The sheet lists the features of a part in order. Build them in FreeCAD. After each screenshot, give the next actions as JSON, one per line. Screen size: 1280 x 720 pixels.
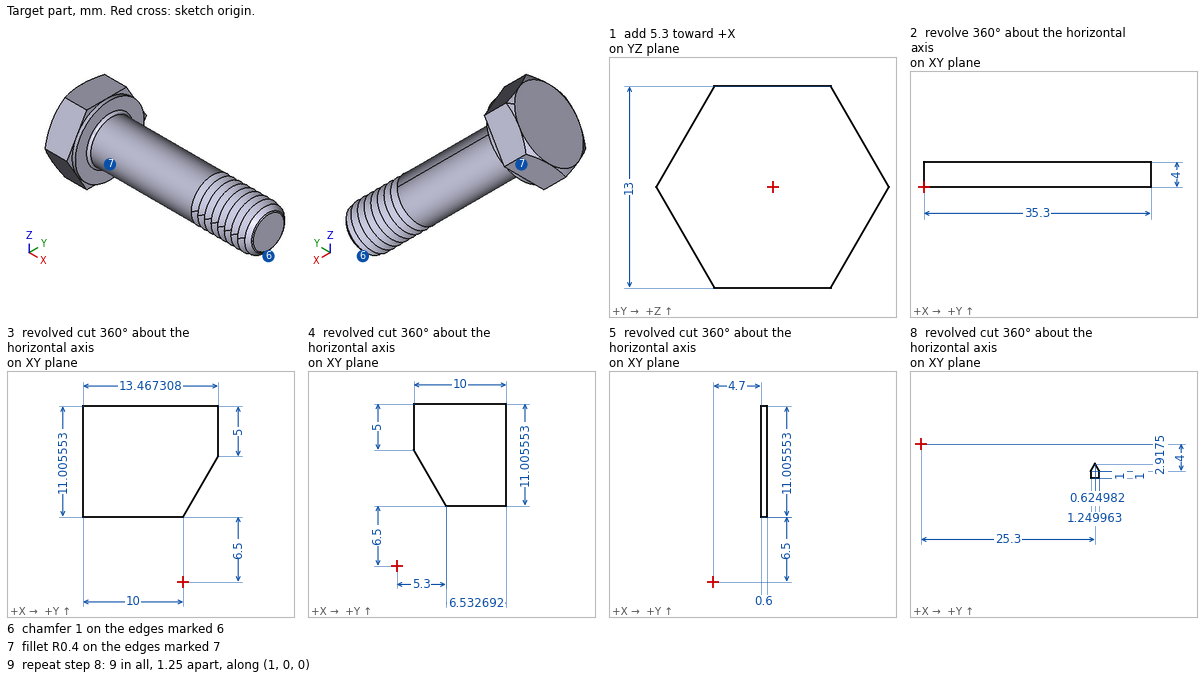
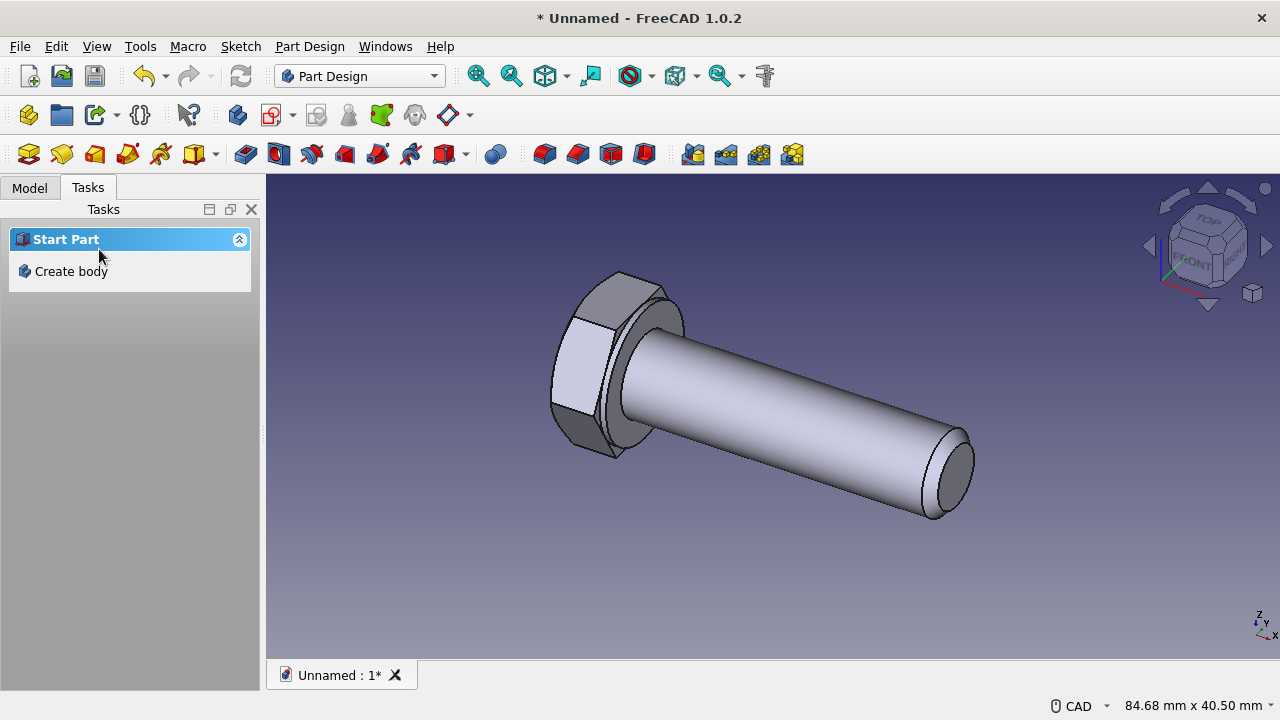
{"action": "key", "text": "0"}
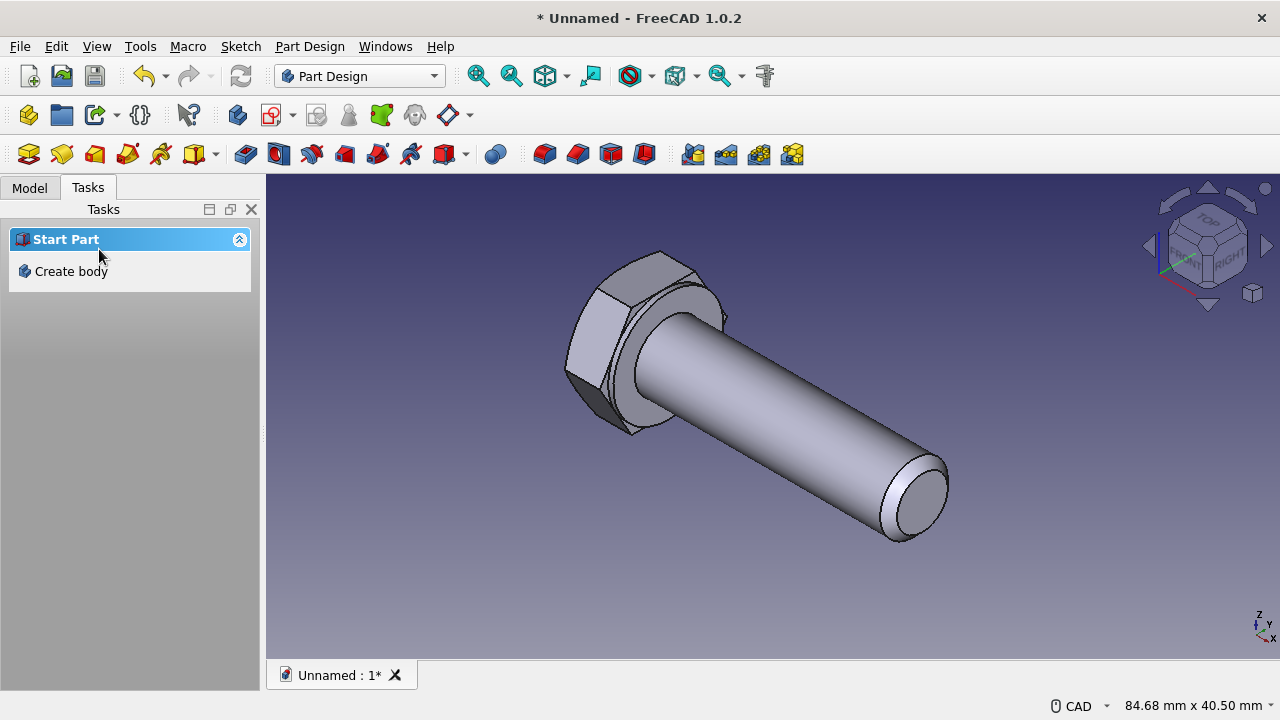
{"action": "key", "text": "2"}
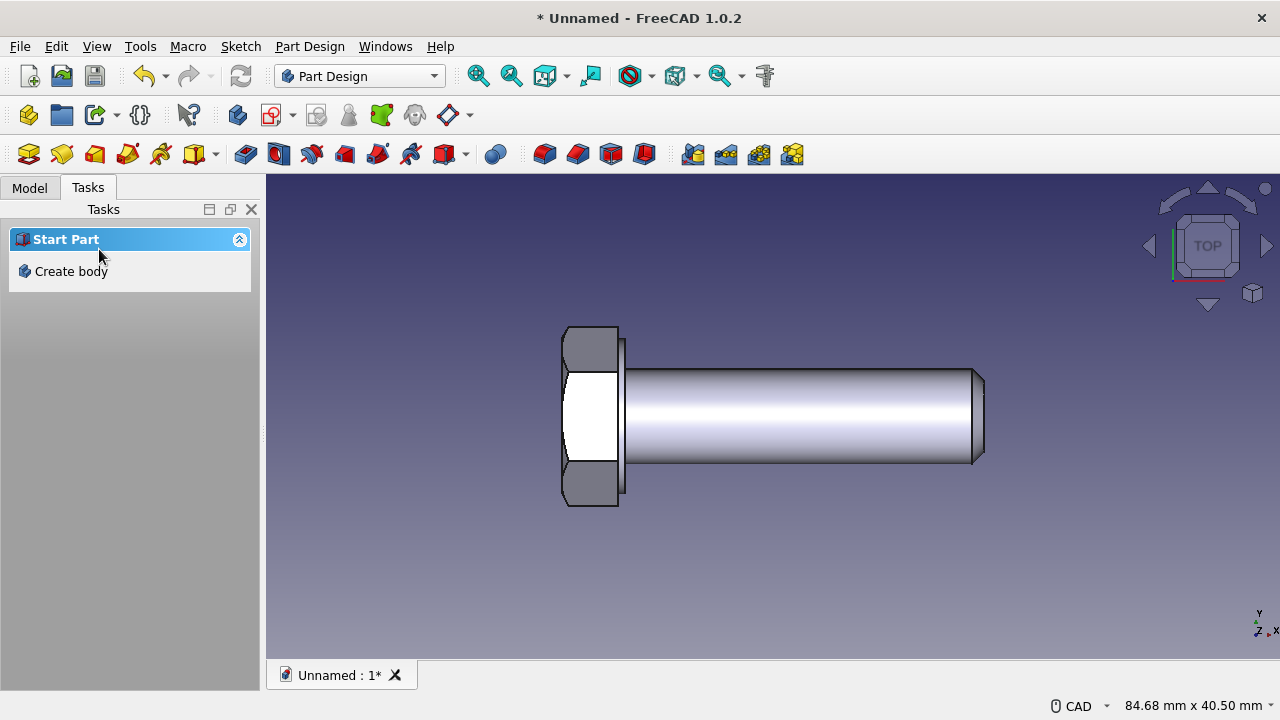
{"action": "left_click", "coordinate": [479, 76]}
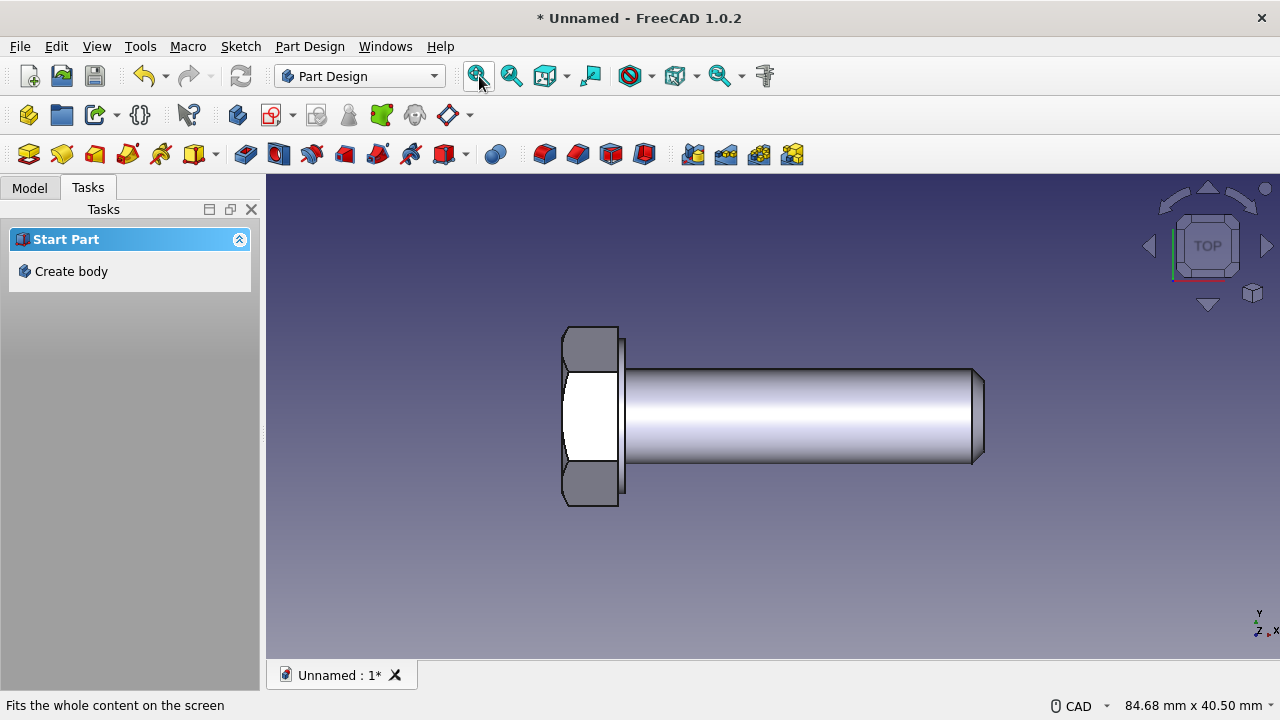
{"action": "key", "text": "1"}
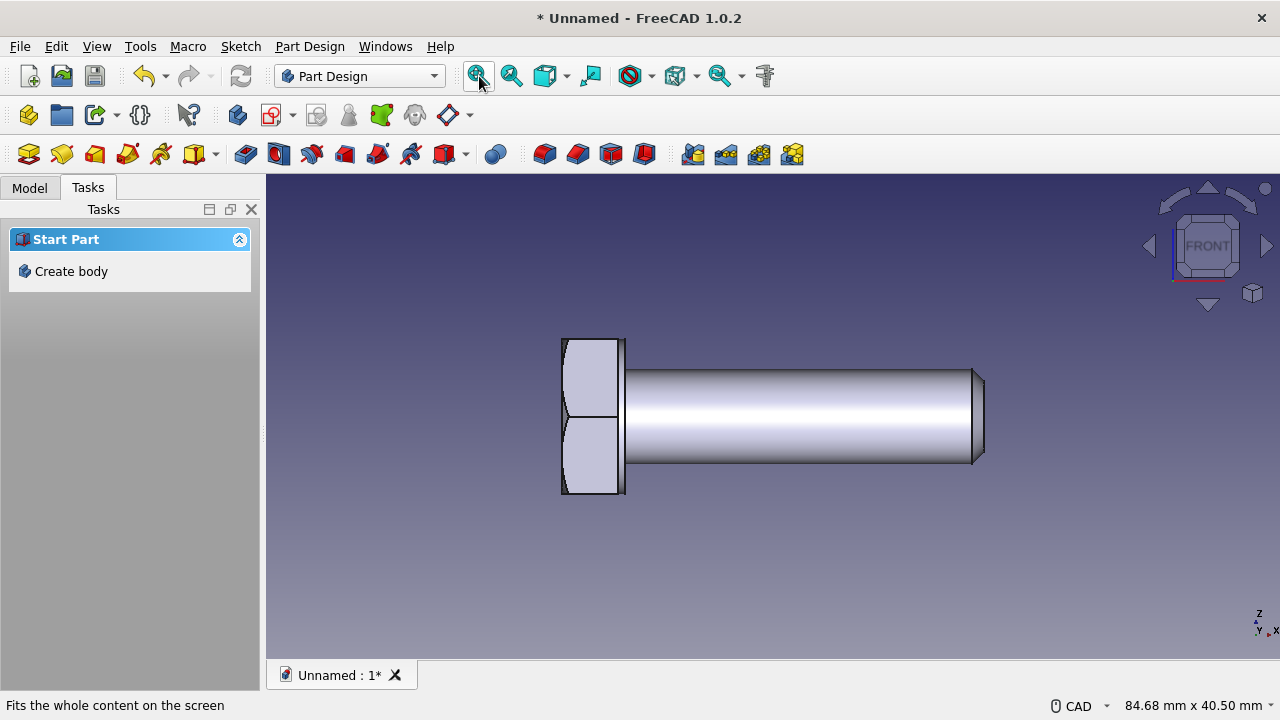
{"action": "left_click", "coordinate": [479, 76]}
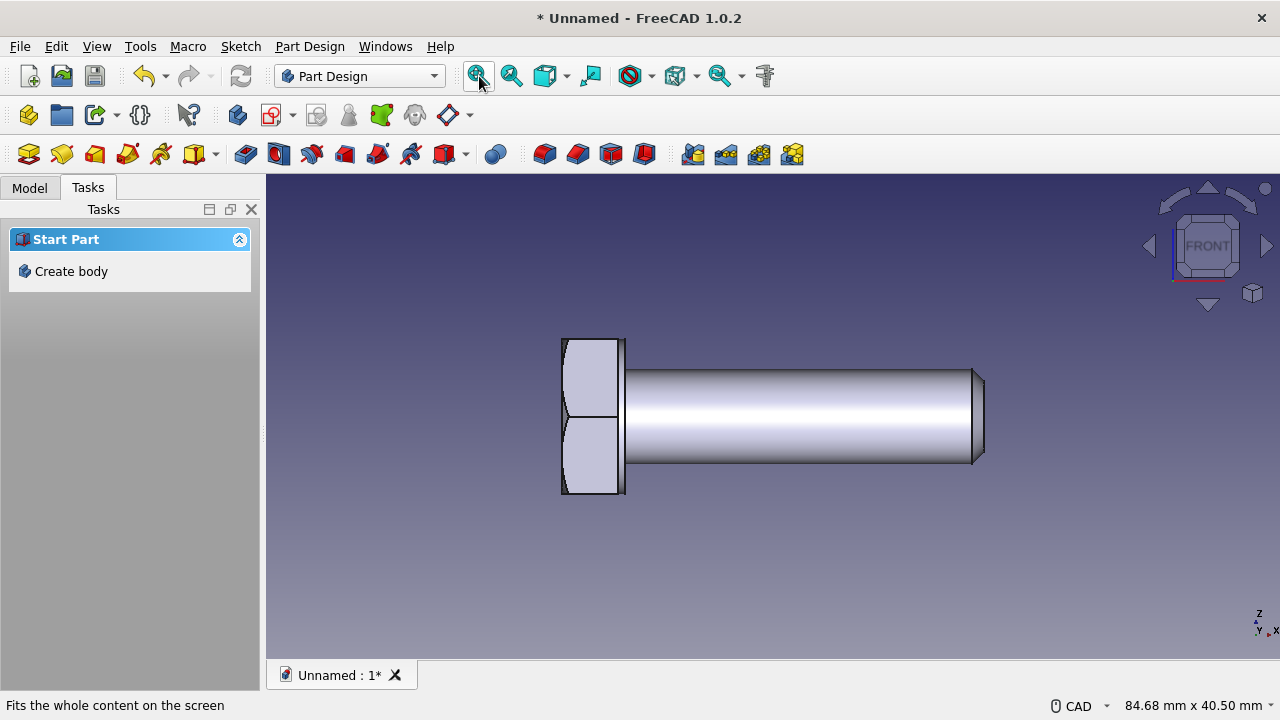
{"action": "key", "text": "3"}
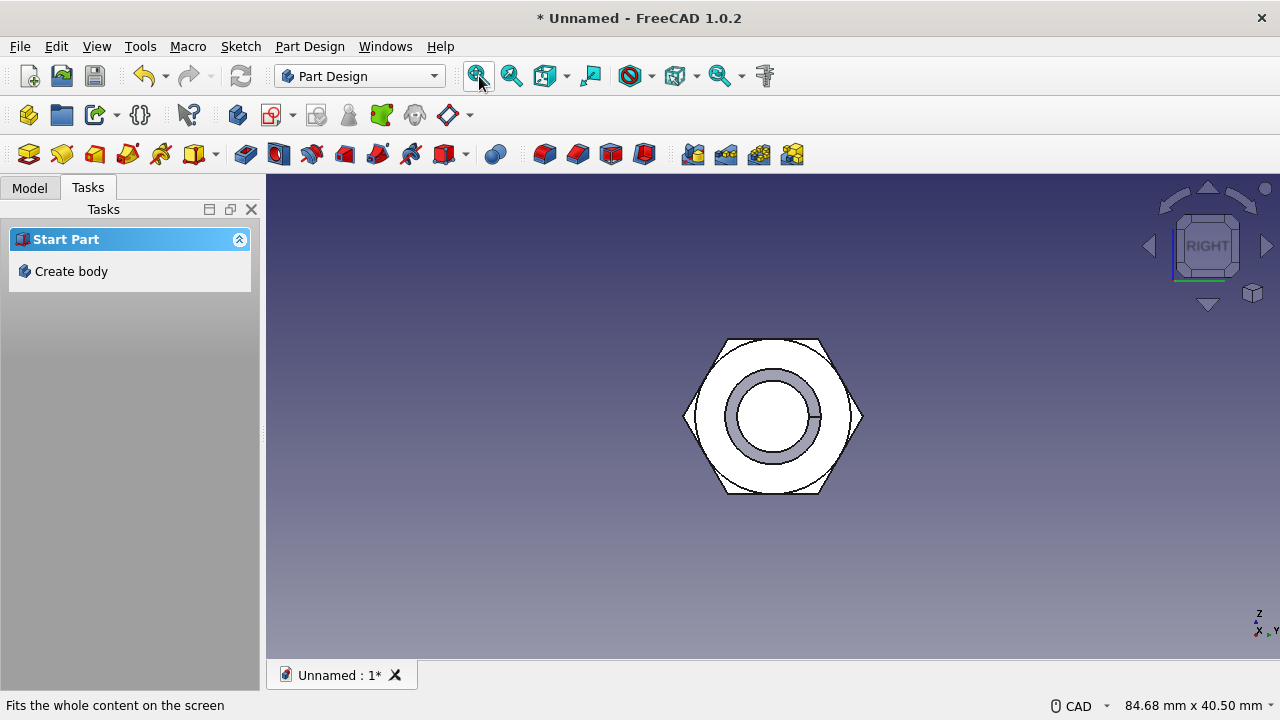
{"action": "left_click", "coordinate": [479, 76]}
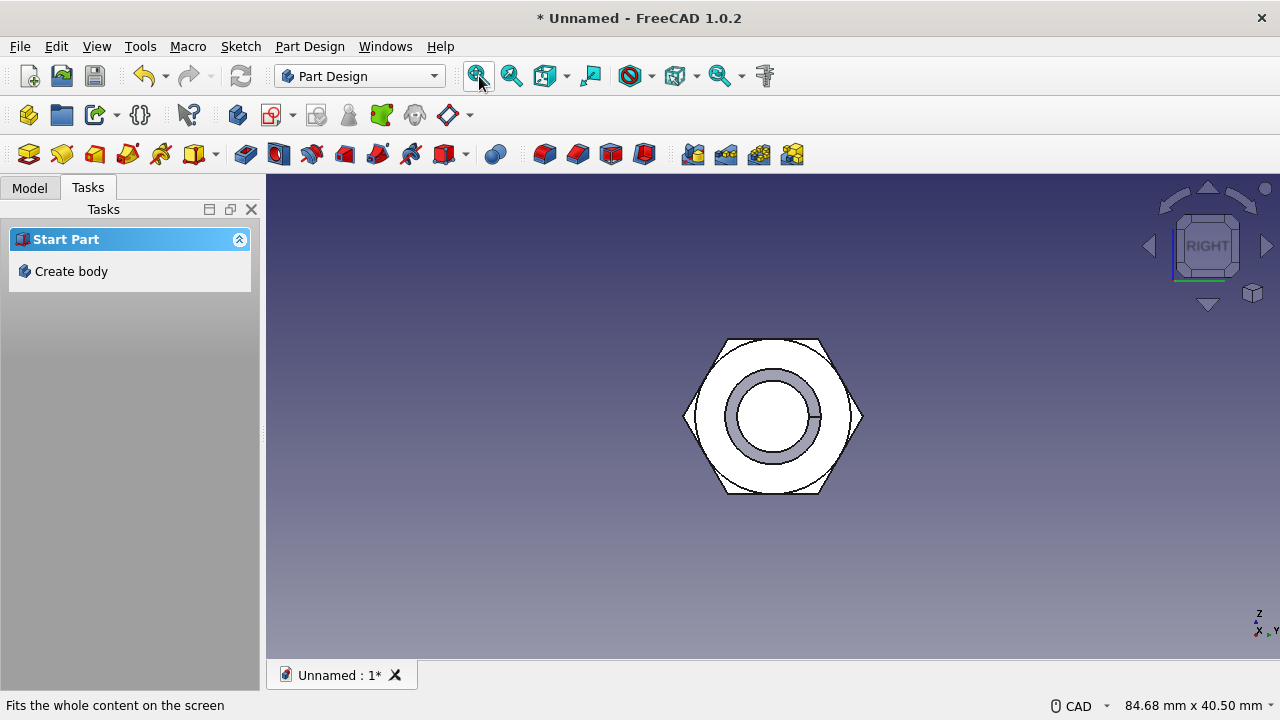
{"action": "key", "text": "5"}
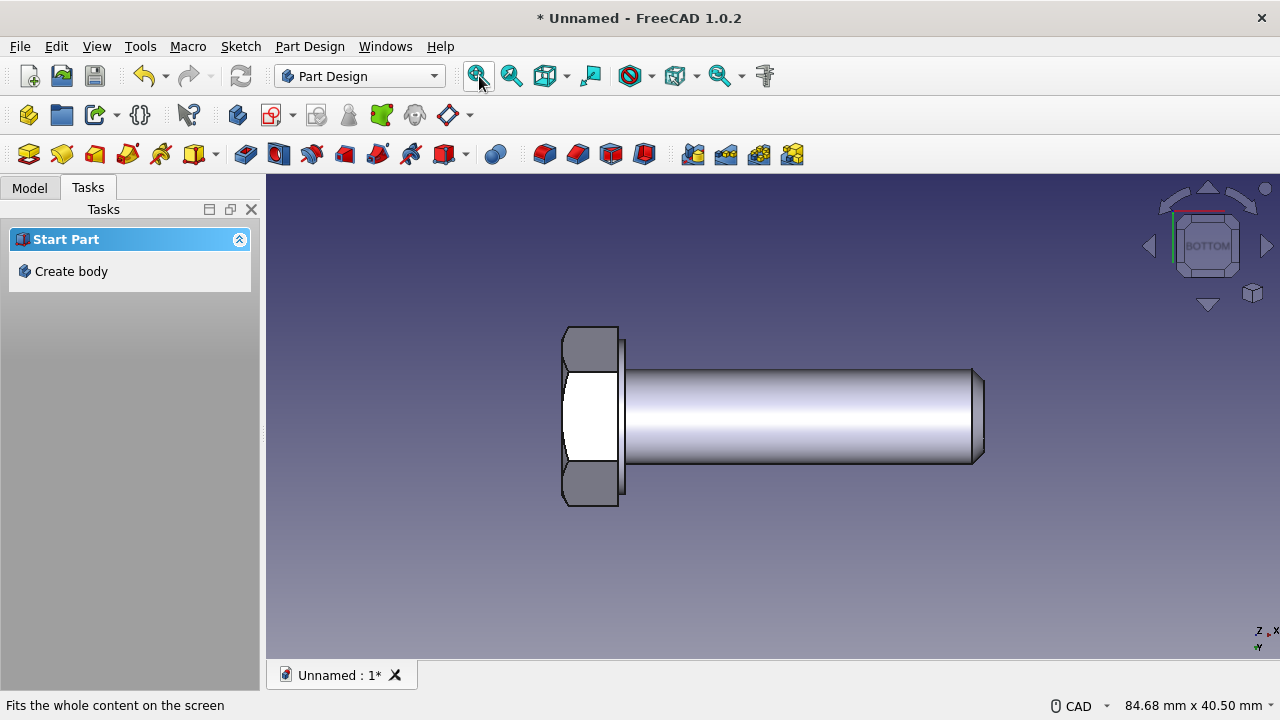
{"action": "key", "text": "v f"}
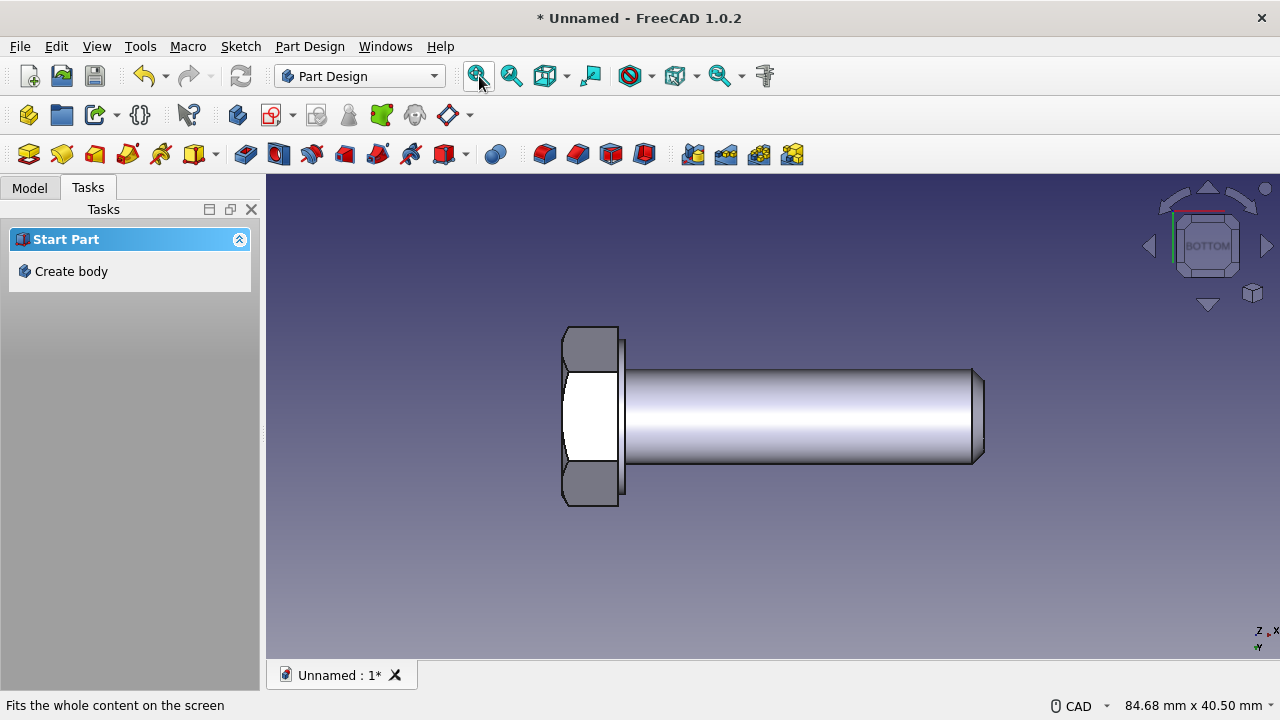
{"action": "key", "text": "4"}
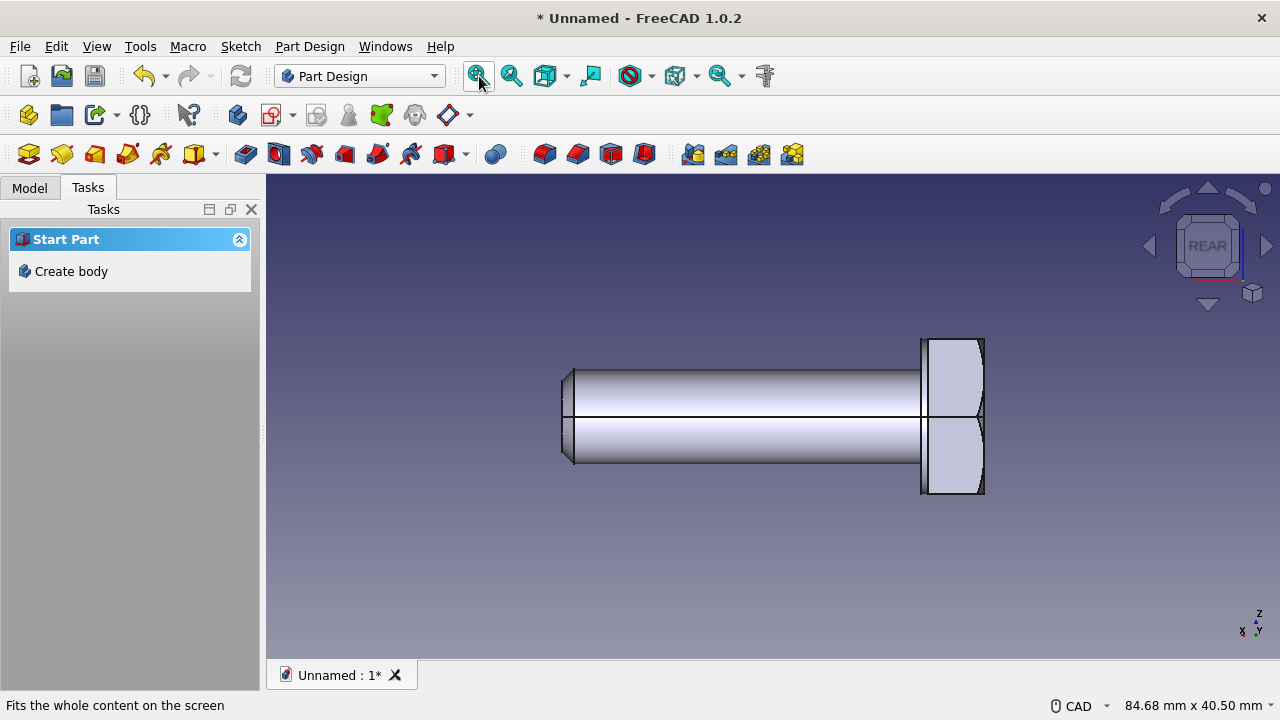
{"action": "left_click", "coordinate": [479, 76]}